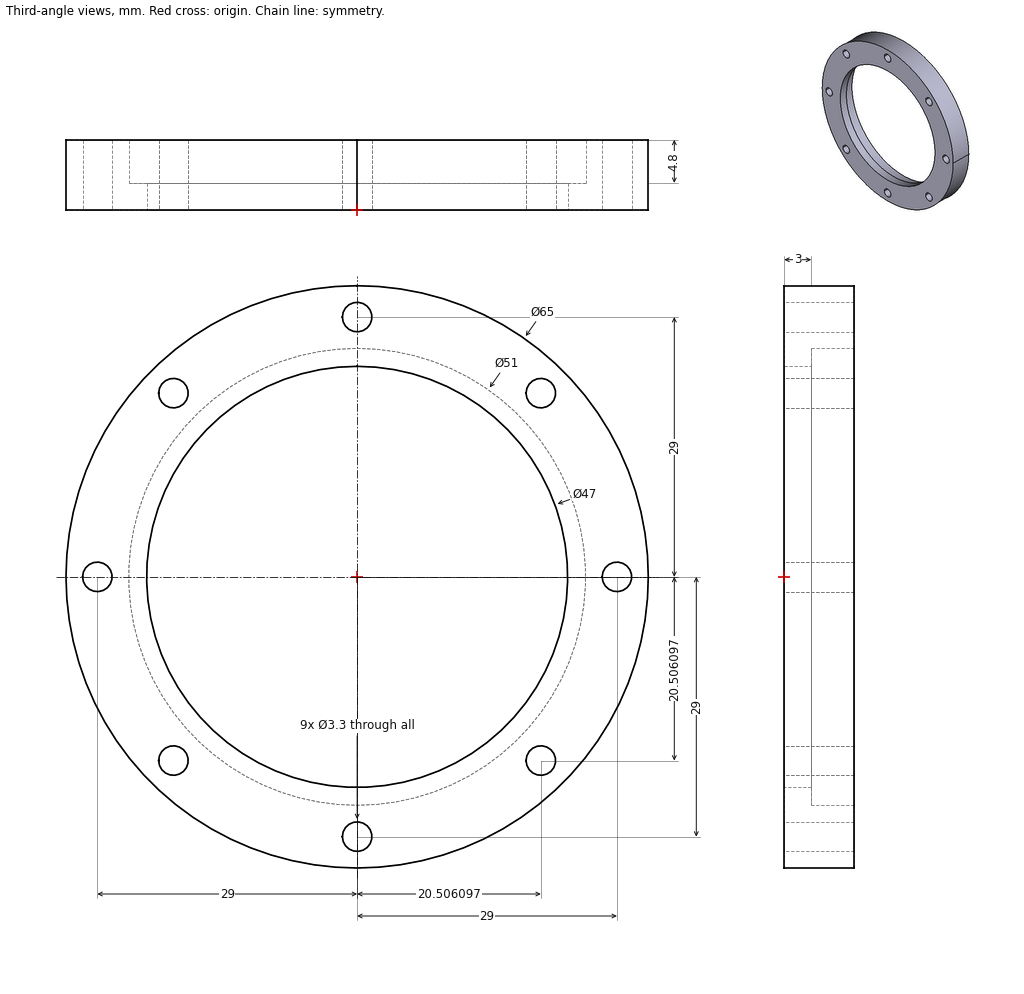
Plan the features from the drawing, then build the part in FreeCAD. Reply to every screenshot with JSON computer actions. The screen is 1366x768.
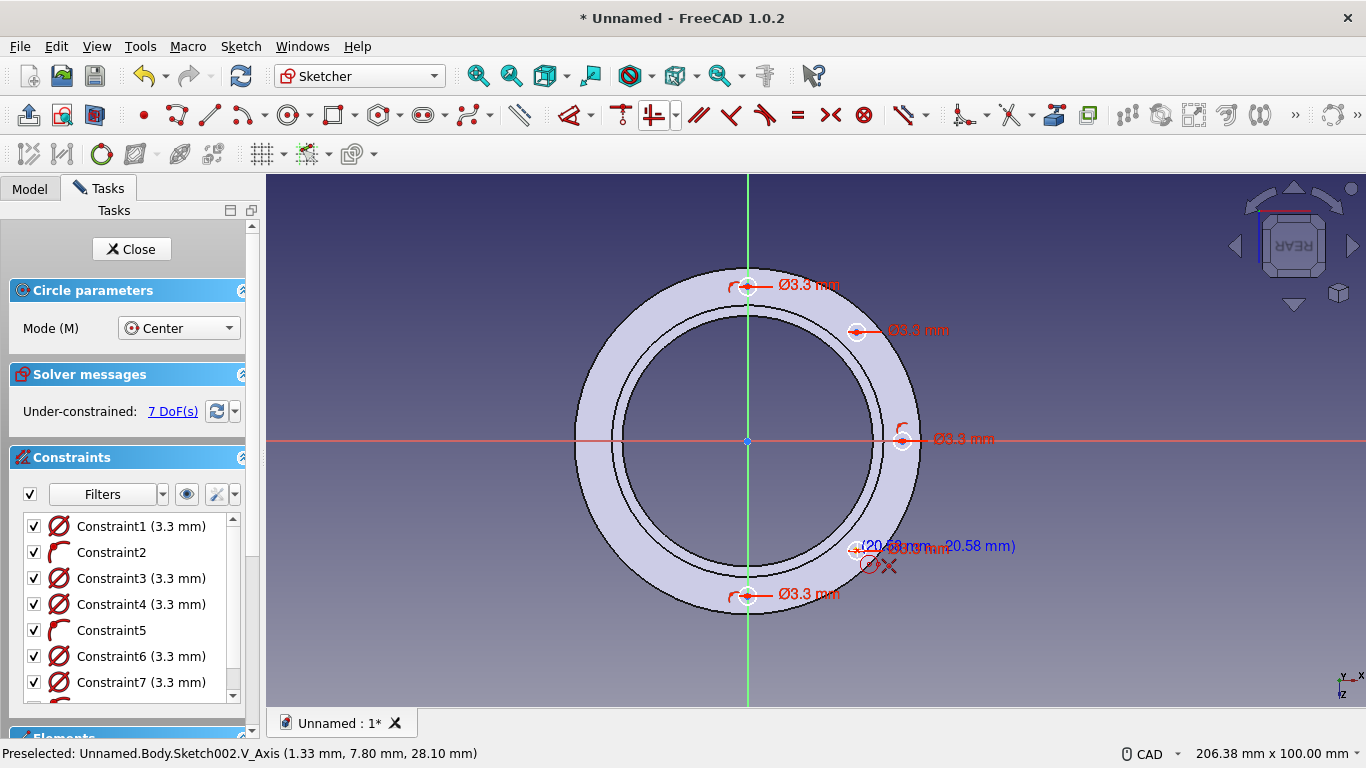
{"action": "scroll", "coordinate": [638, 550], "scroll_direction": "up", "scroll_amount": 5}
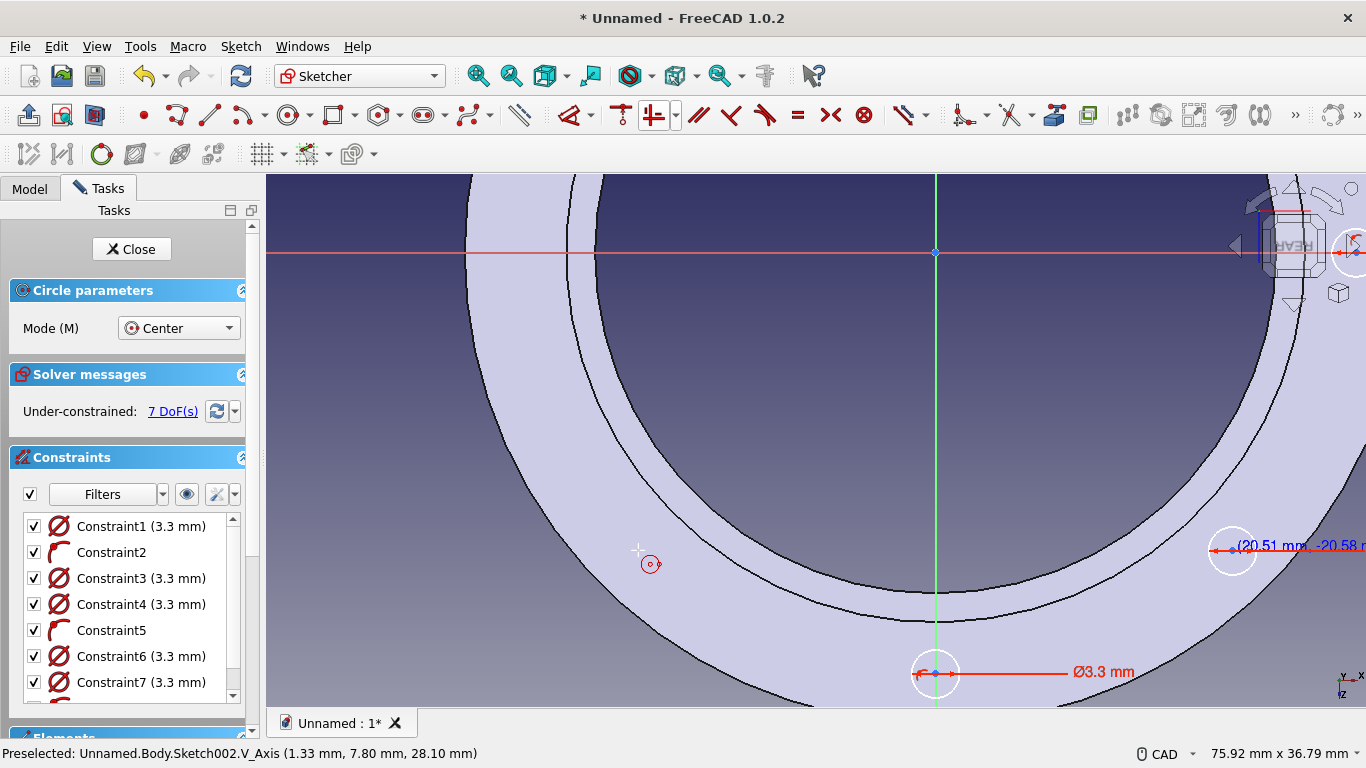
{"action": "left_click", "coordinate": [638, 550]}
{"action": "mouse_move", "coordinate": [655, 533]}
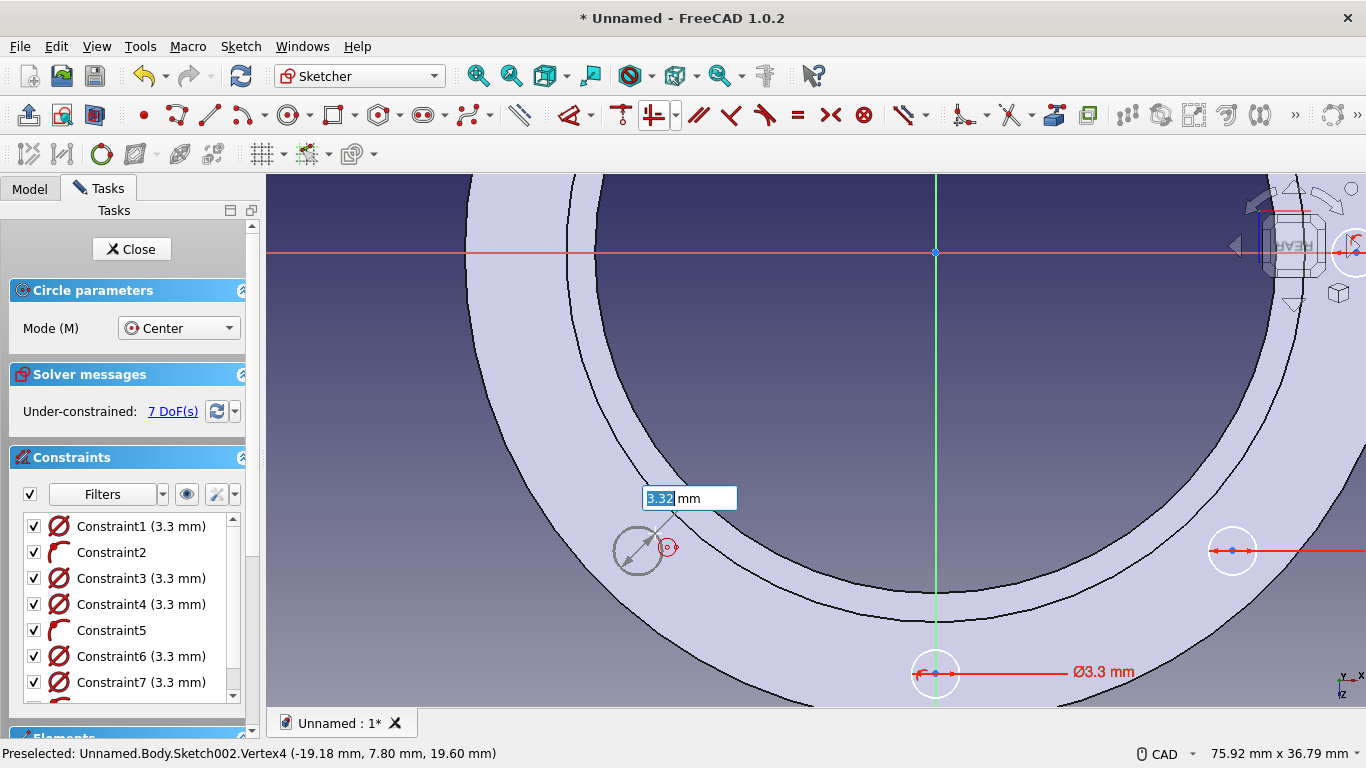
{"action": "type", "text": "3.3"}
{"action": "key", "text": "Return"}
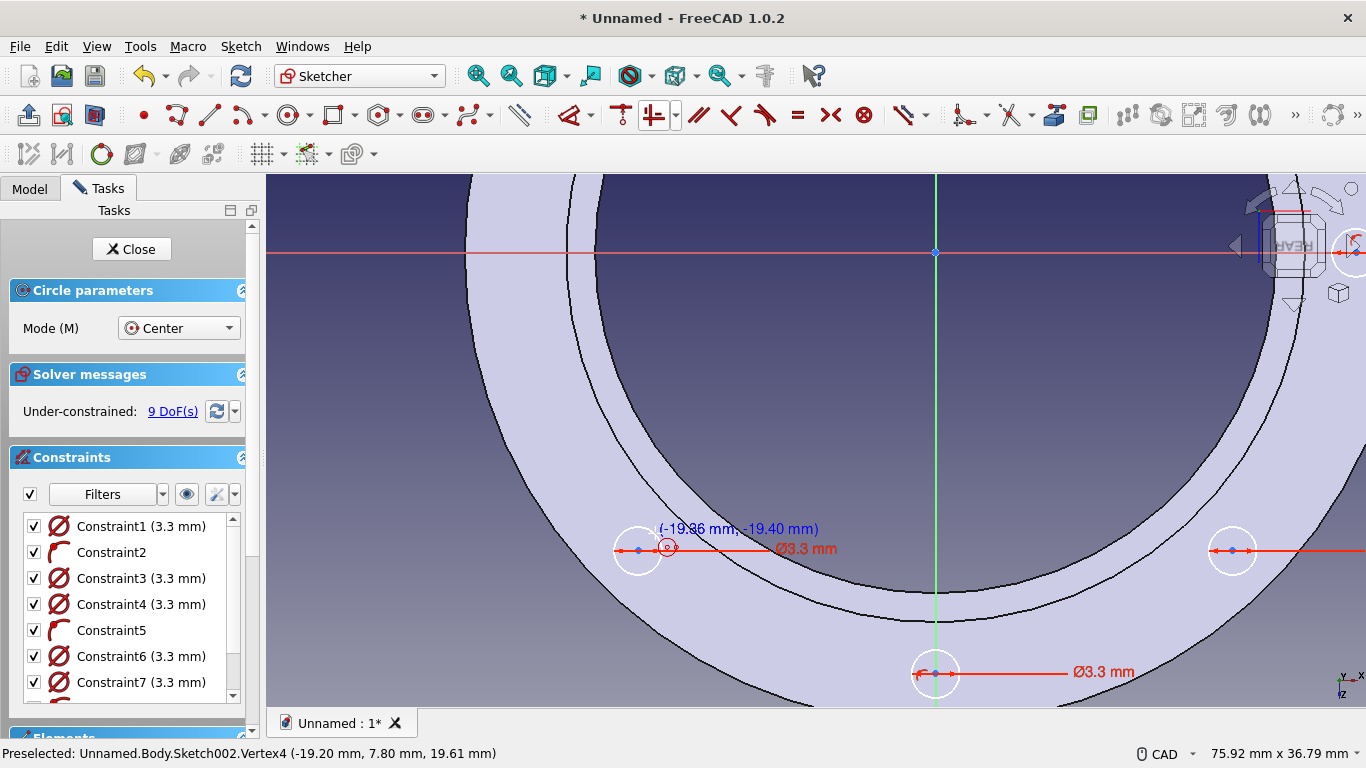
{"action": "left_click", "coordinate": [515, 253]}
{"action": "mouse_move", "coordinate": [532, 236]}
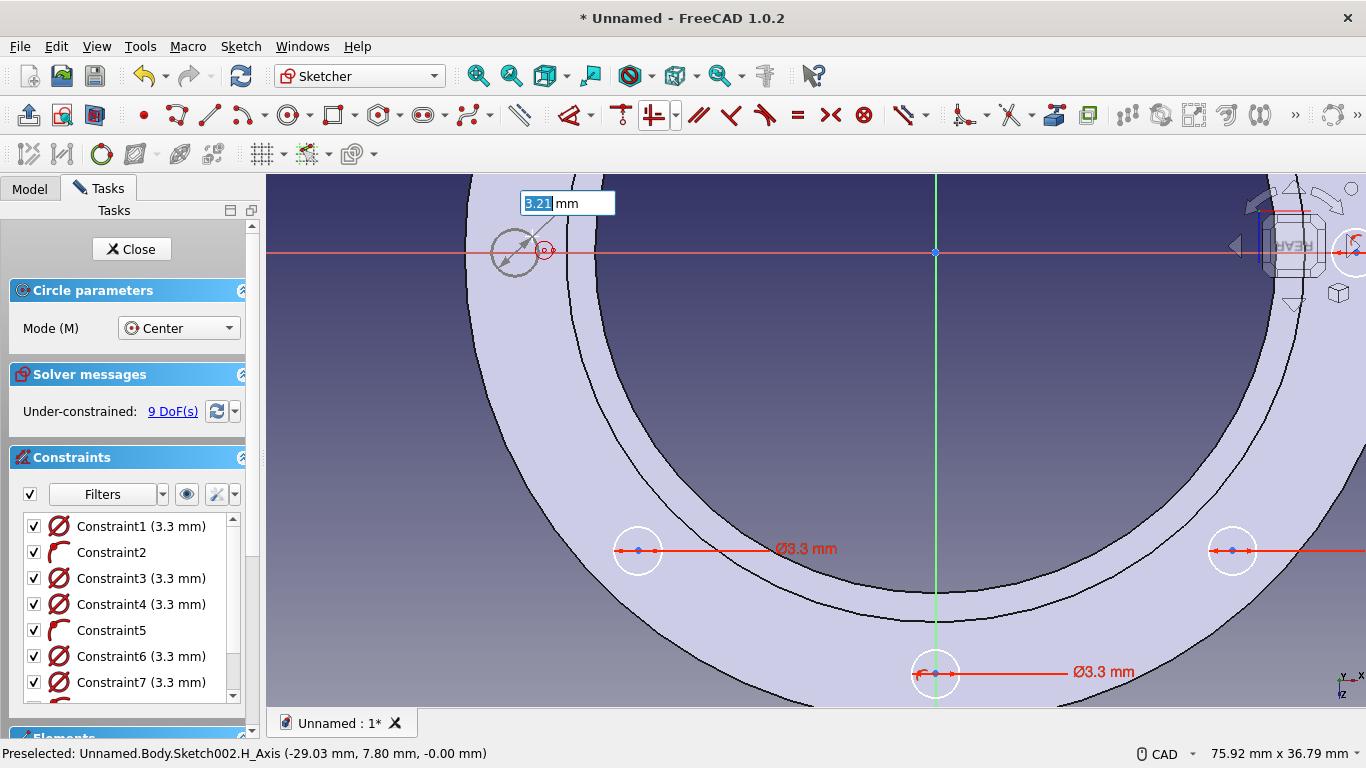
{"action": "type", "text": "3.3"}
{"action": "key", "text": "Return"}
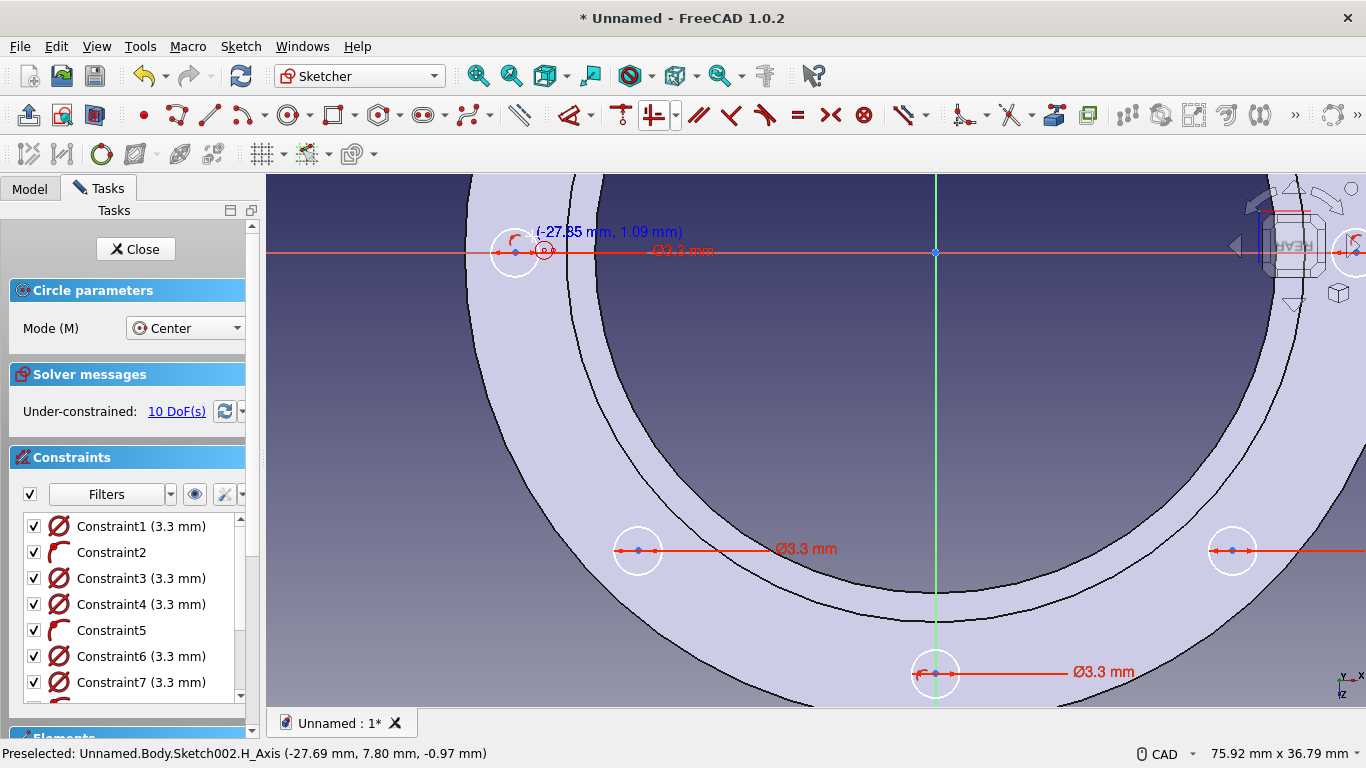
{"action": "scroll", "coordinate": [638, 550], "scroll_direction": "down", "scroll_amount": 5}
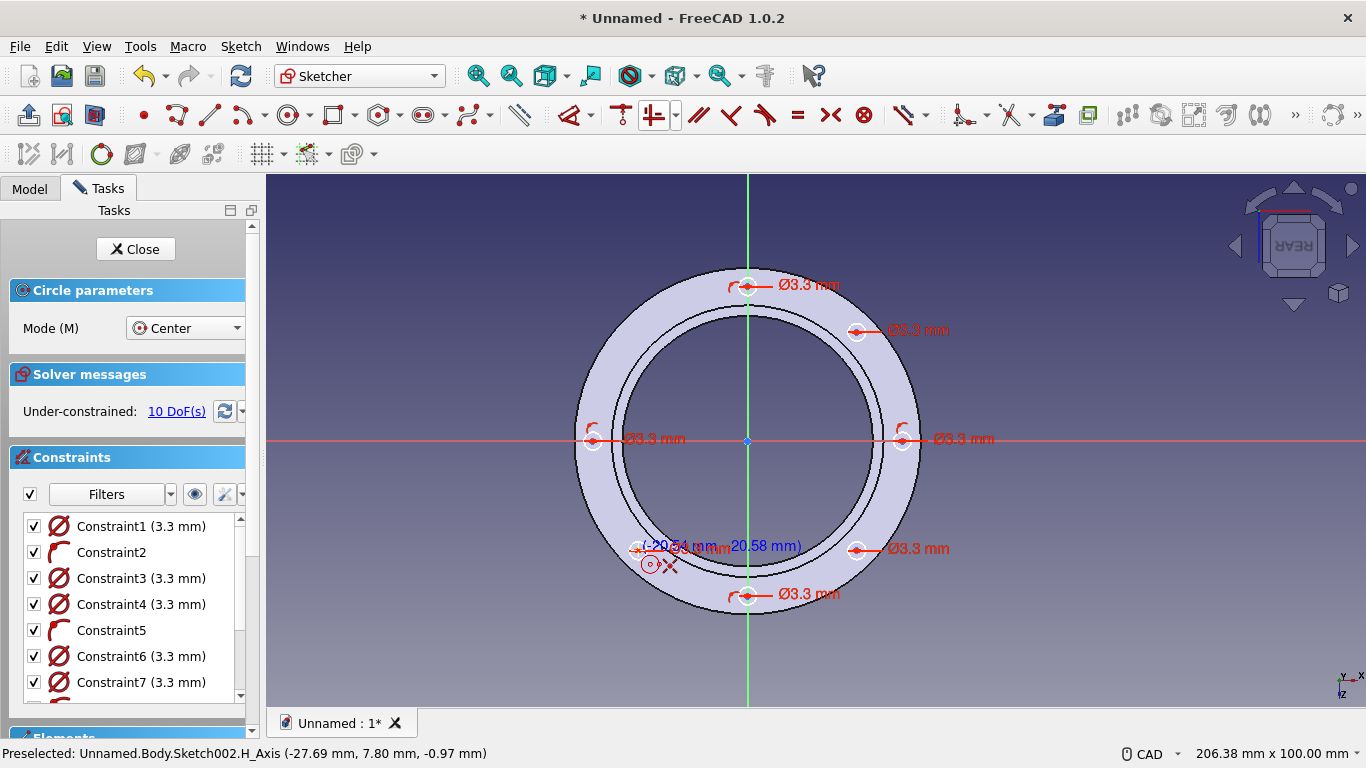
{"action": "scroll", "coordinate": [638, 332], "scroll_direction": "up", "scroll_amount": 5}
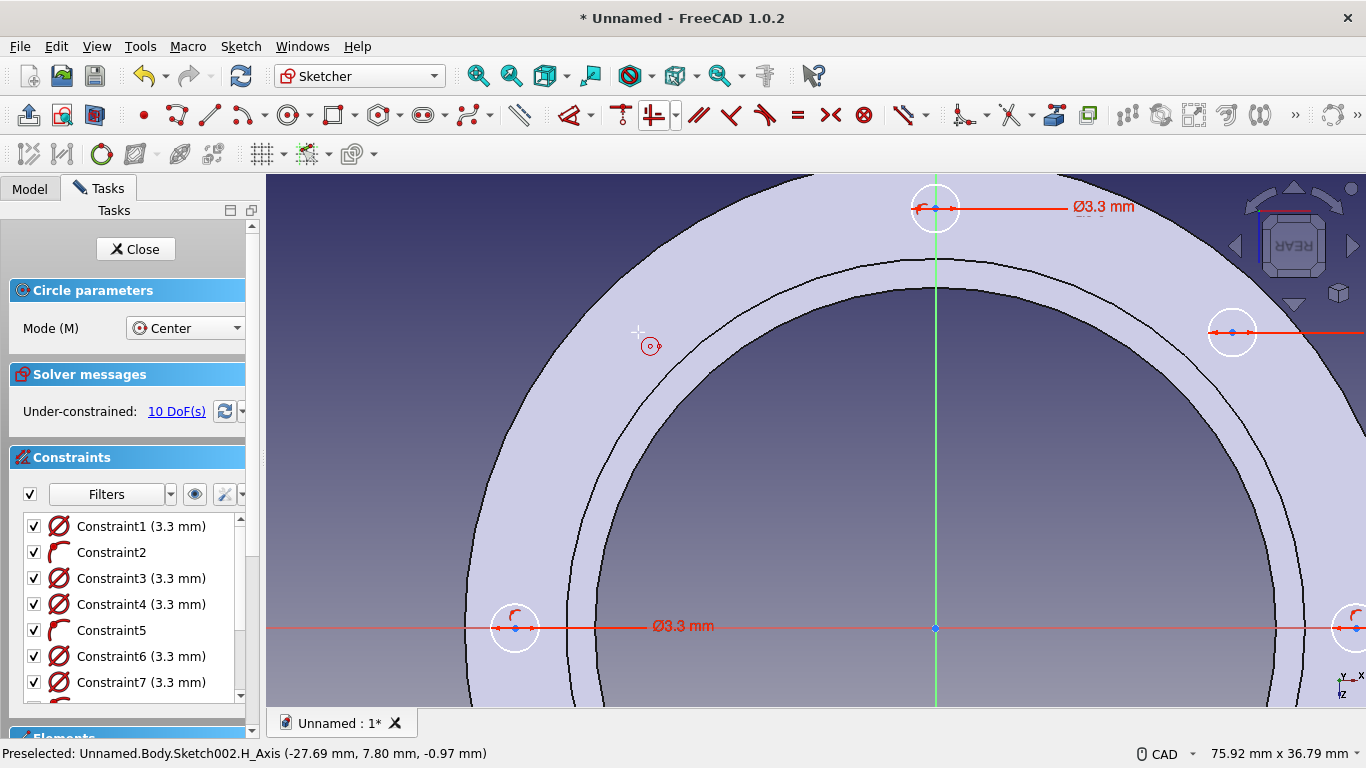
{"action": "left_click", "coordinate": [638, 331]}
{"action": "mouse_move", "coordinate": [655, 314]}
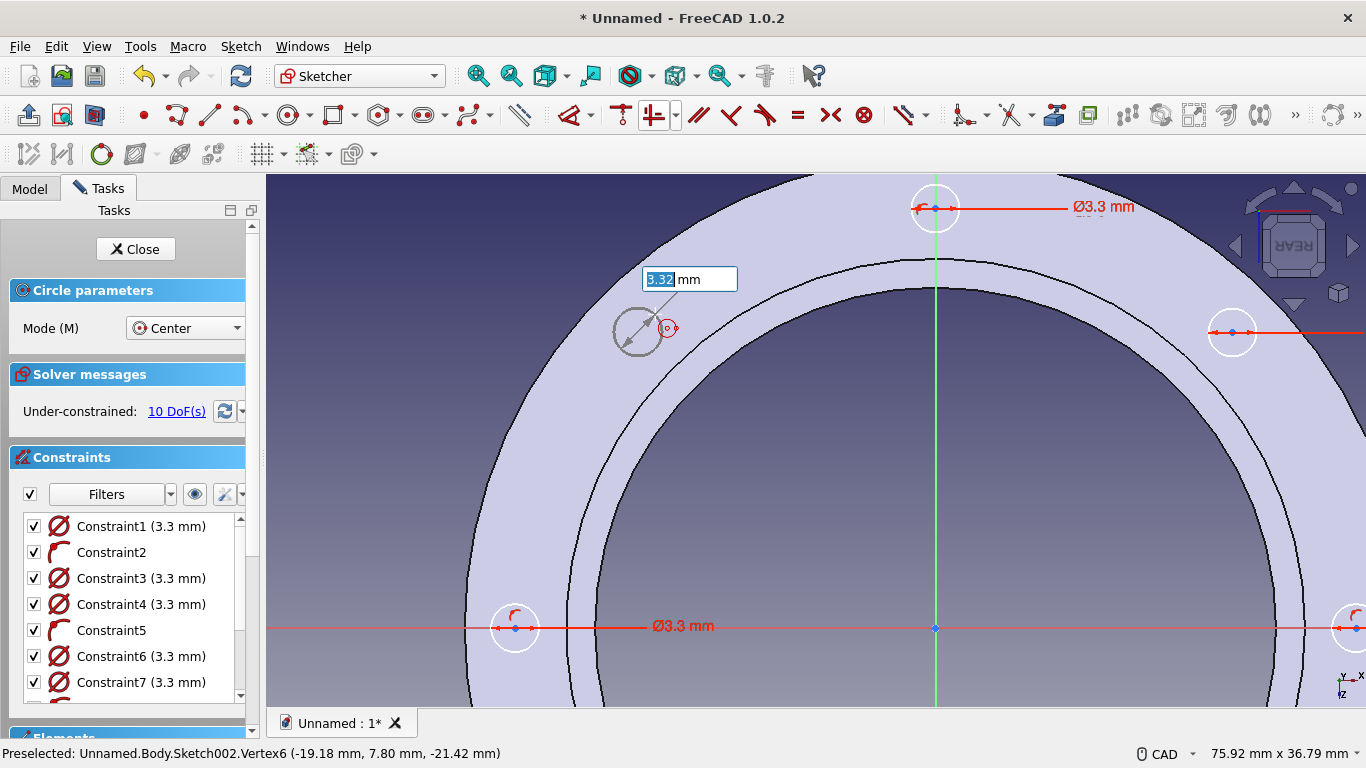
{"action": "type", "text": "3.3"}
{"action": "key", "text": "Return"}